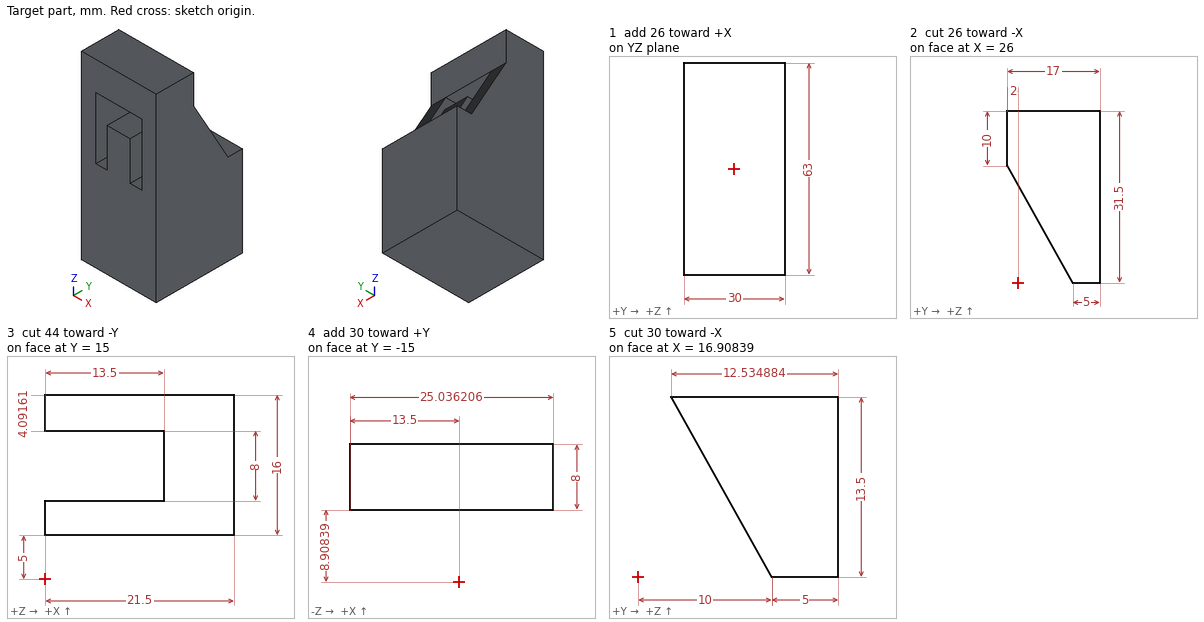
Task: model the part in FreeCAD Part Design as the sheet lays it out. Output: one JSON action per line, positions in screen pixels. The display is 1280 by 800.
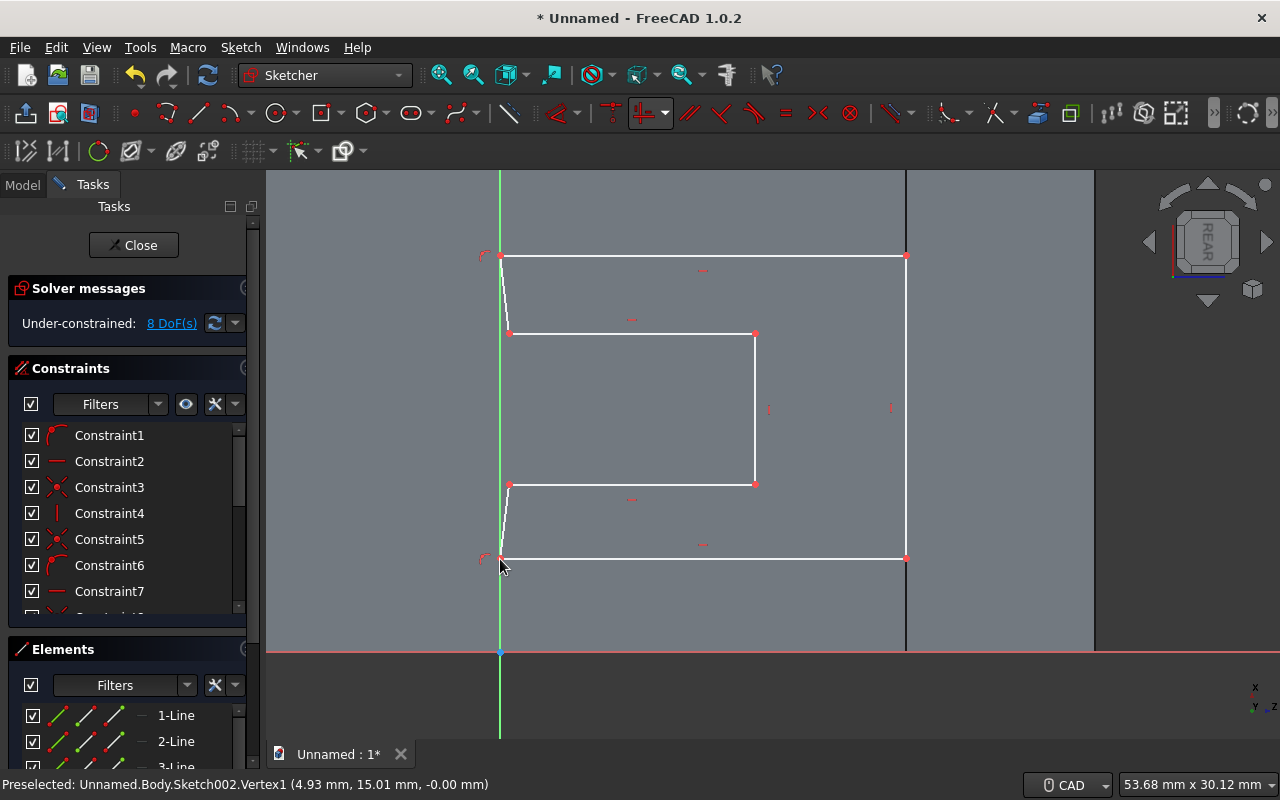
{"action": "left_click", "coordinate": [503, 279]}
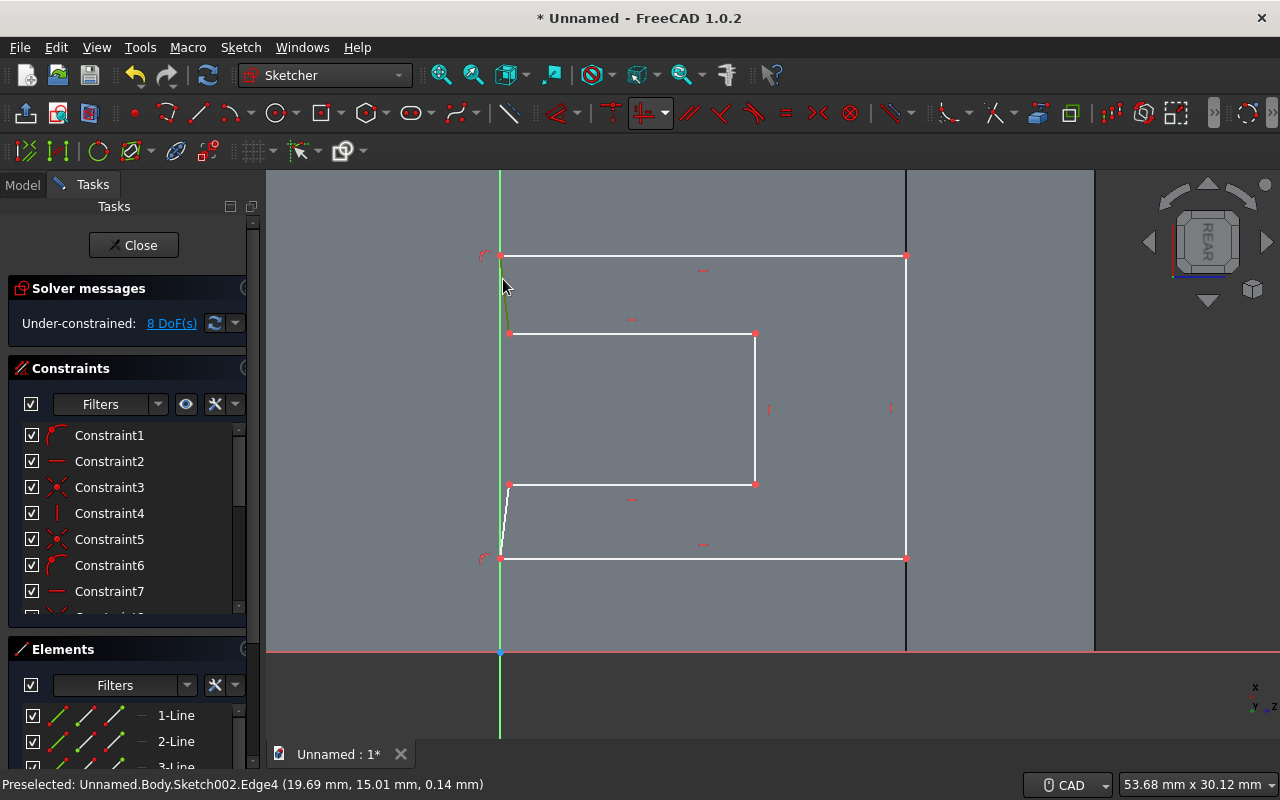
{"action": "key", "text": "v"}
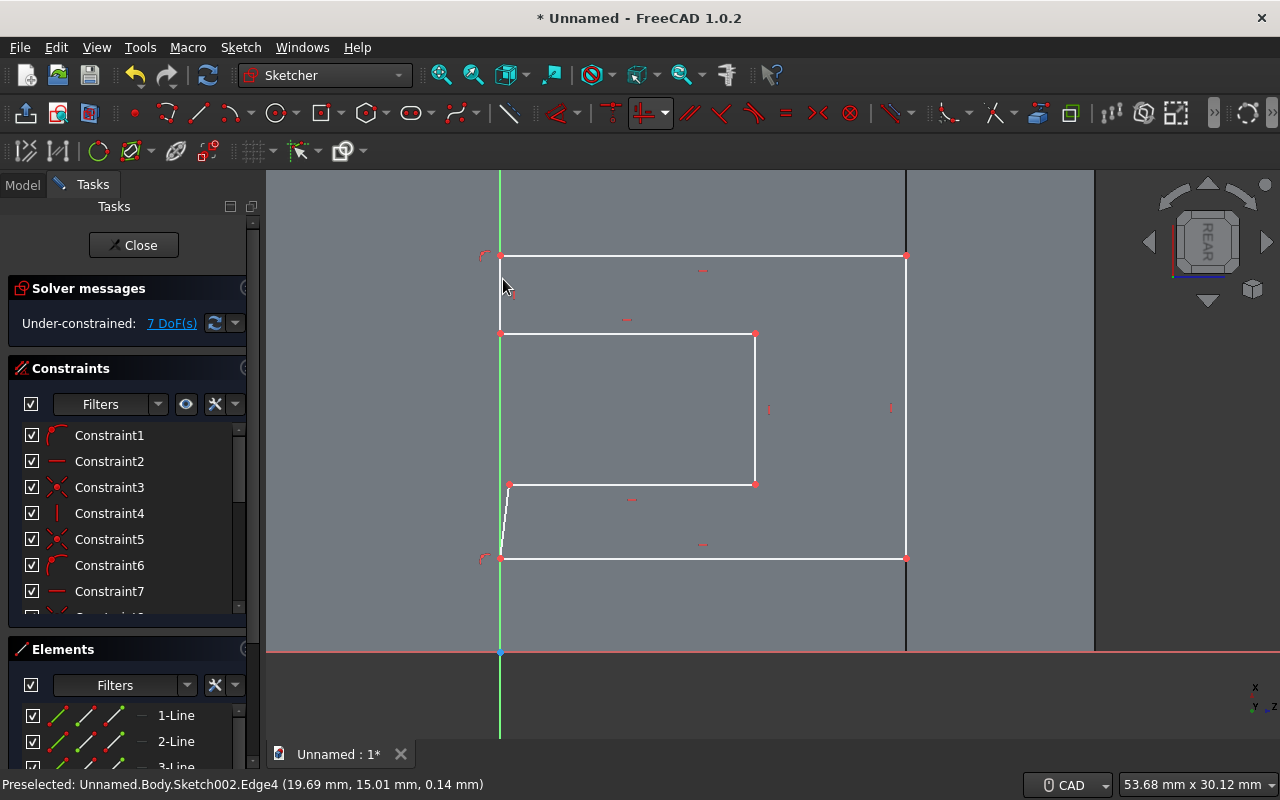
{"action": "left_click", "coordinate": [503, 537]}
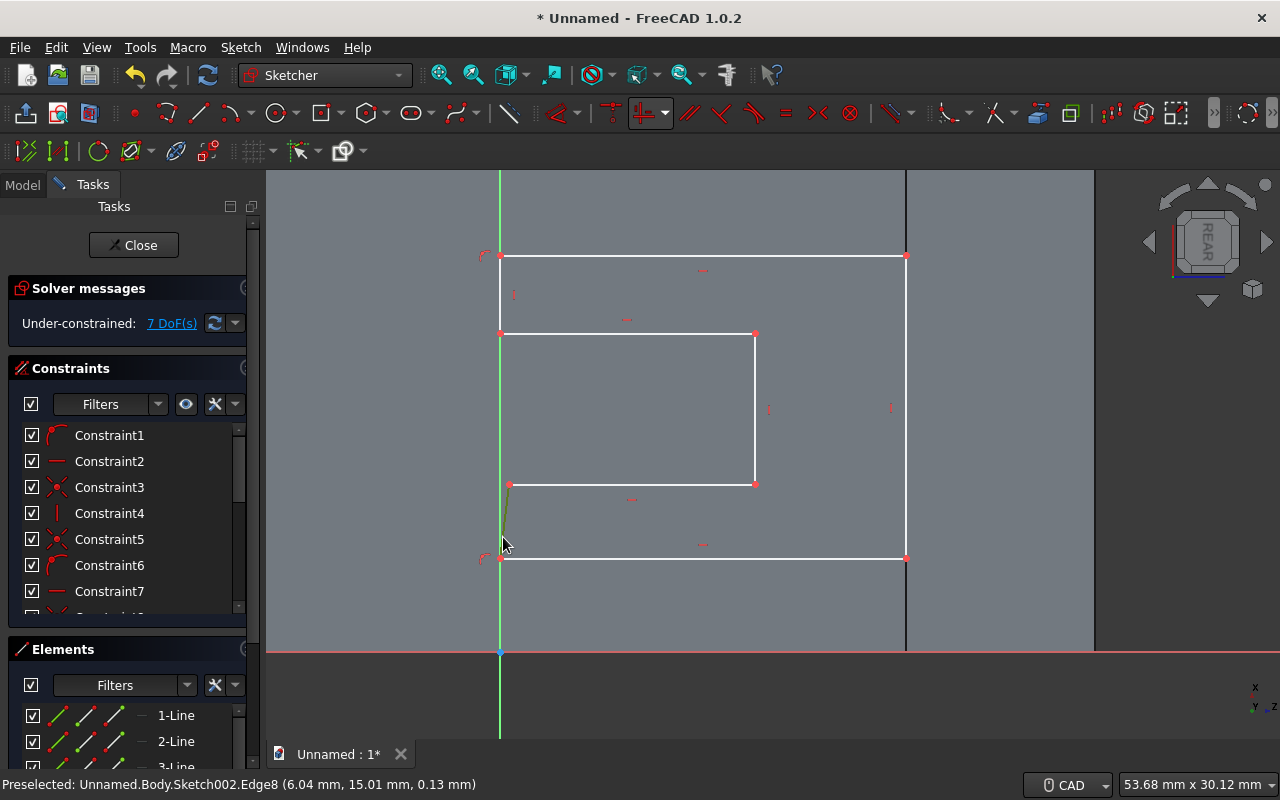
{"action": "key", "text": "v"}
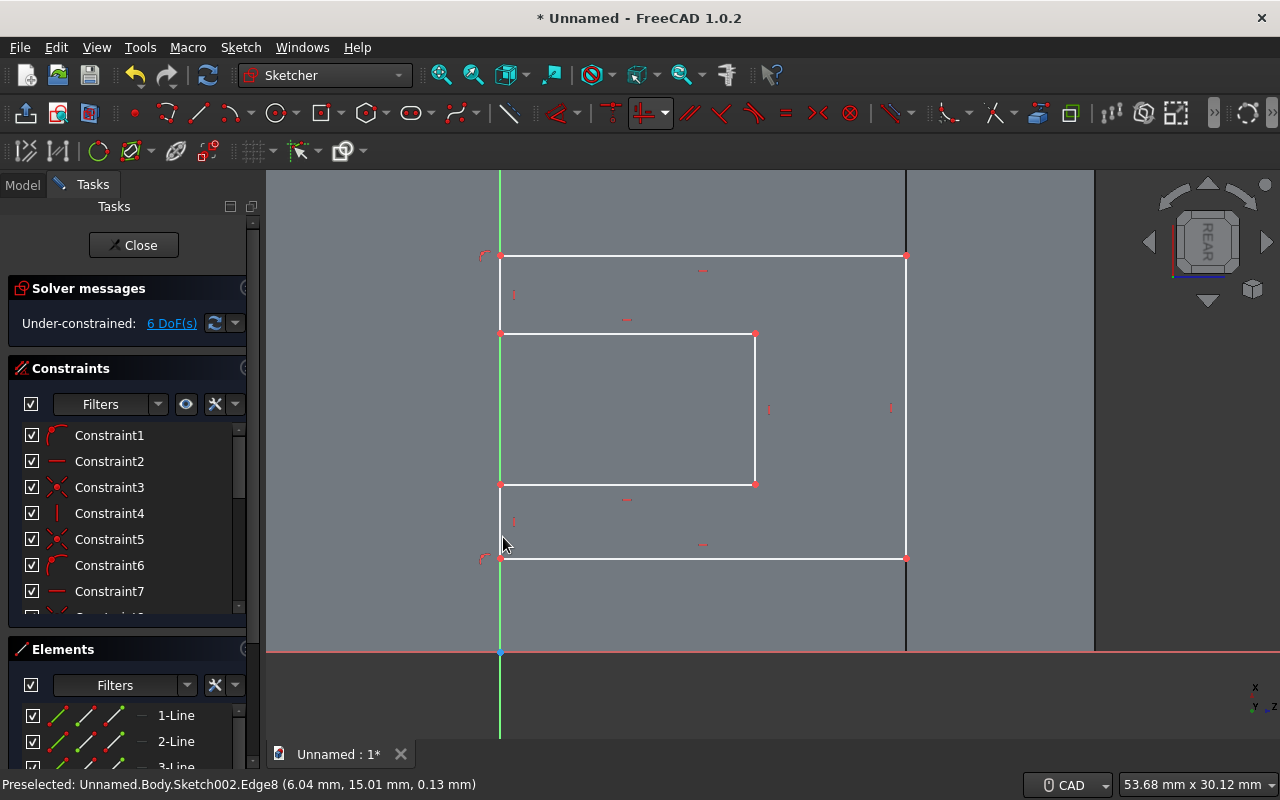
{"action": "key", "text": "d"}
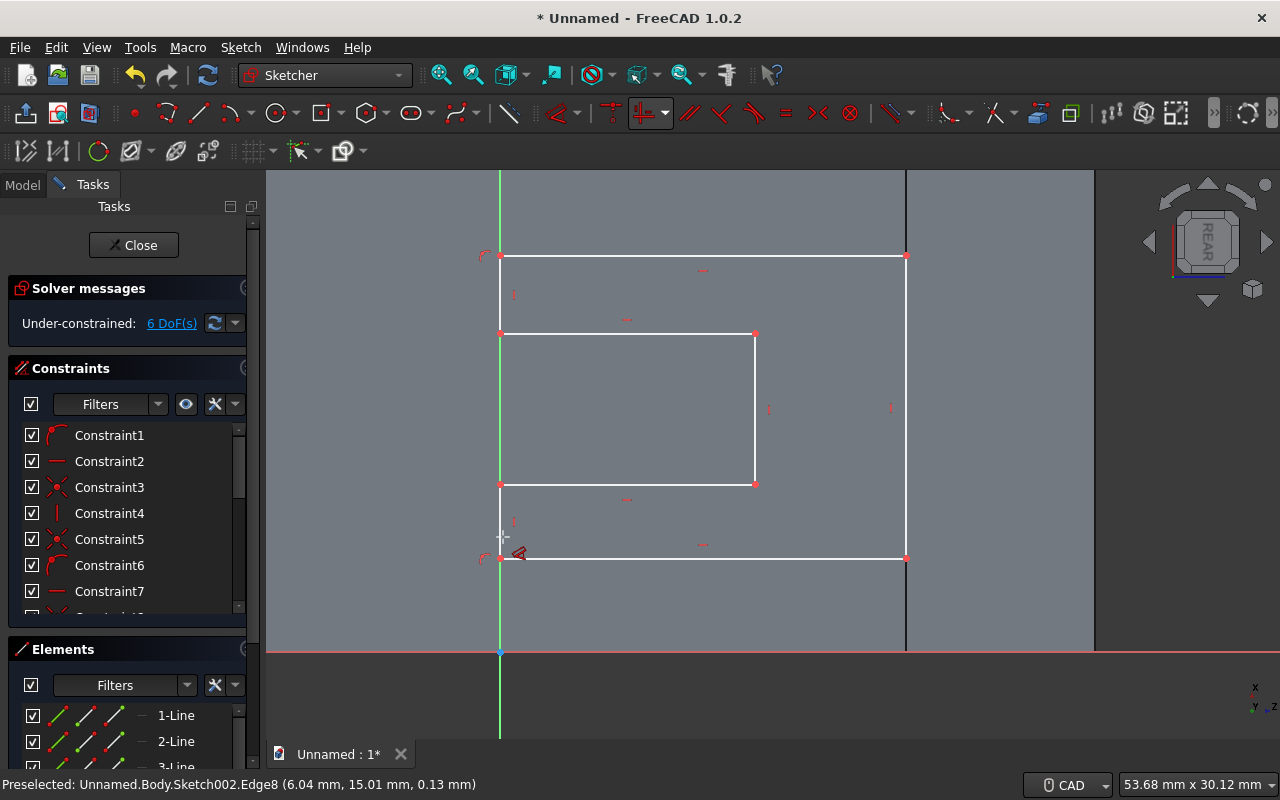
{"action": "left_click", "coordinate": [755, 379]}
{"action": "left_click", "coordinate": [789, 409]}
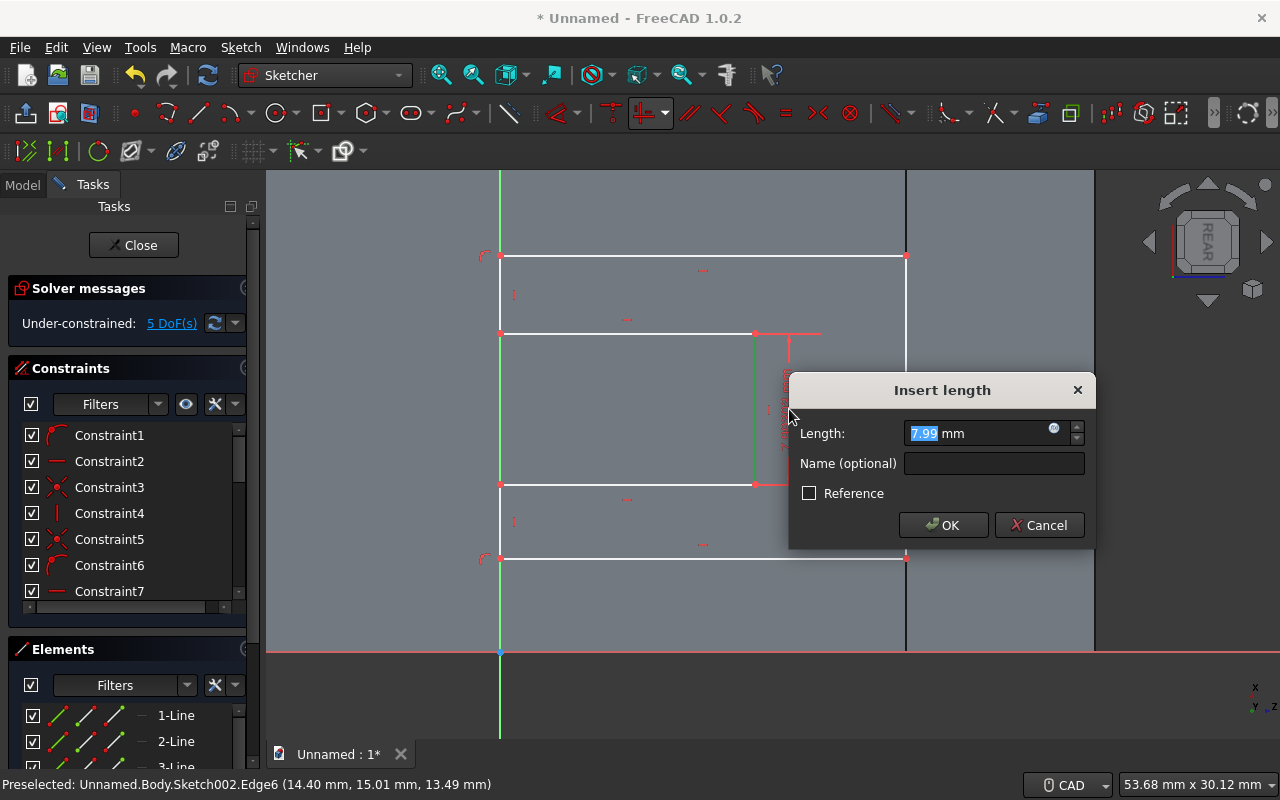
{"action": "type", "text": "8"}
{"action": "key", "text": "Return"}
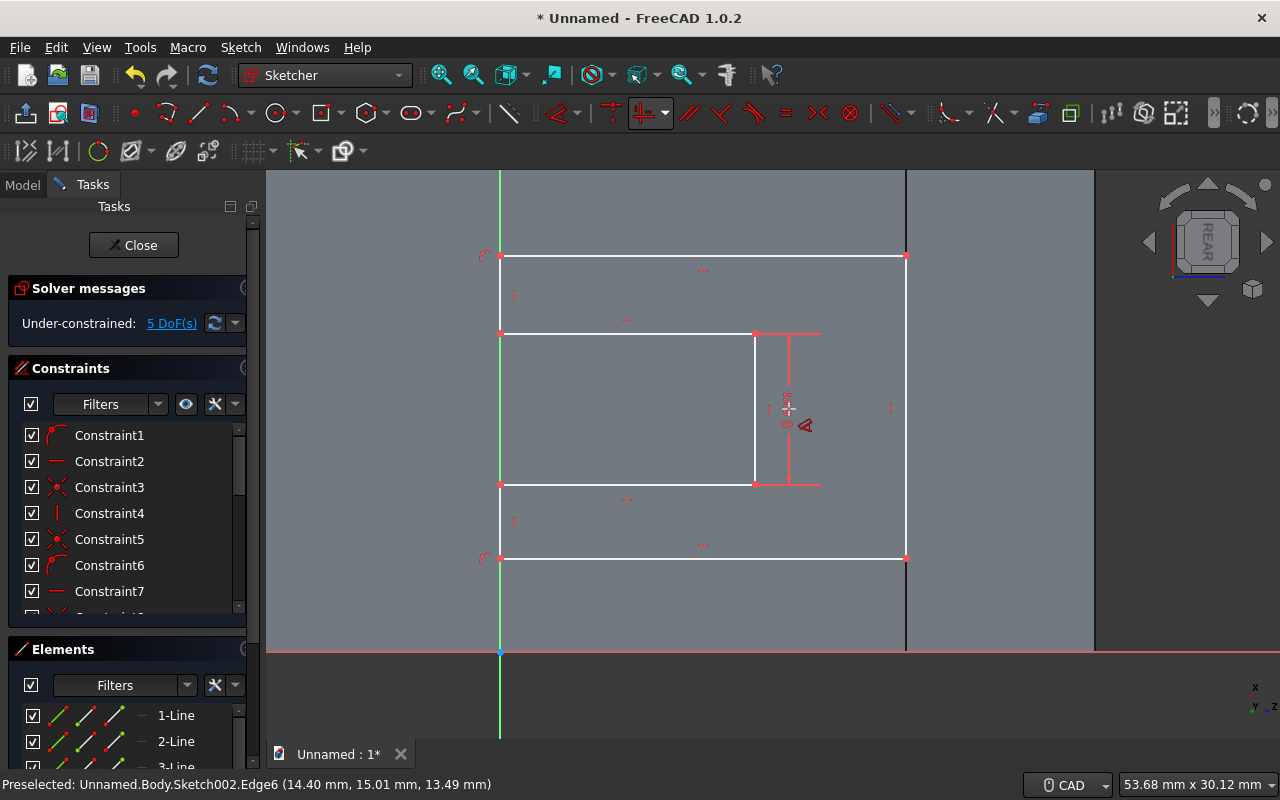
{"action": "left_click", "coordinate": [906, 468]}
{"action": "left_click", "coordinate": [940, 408]}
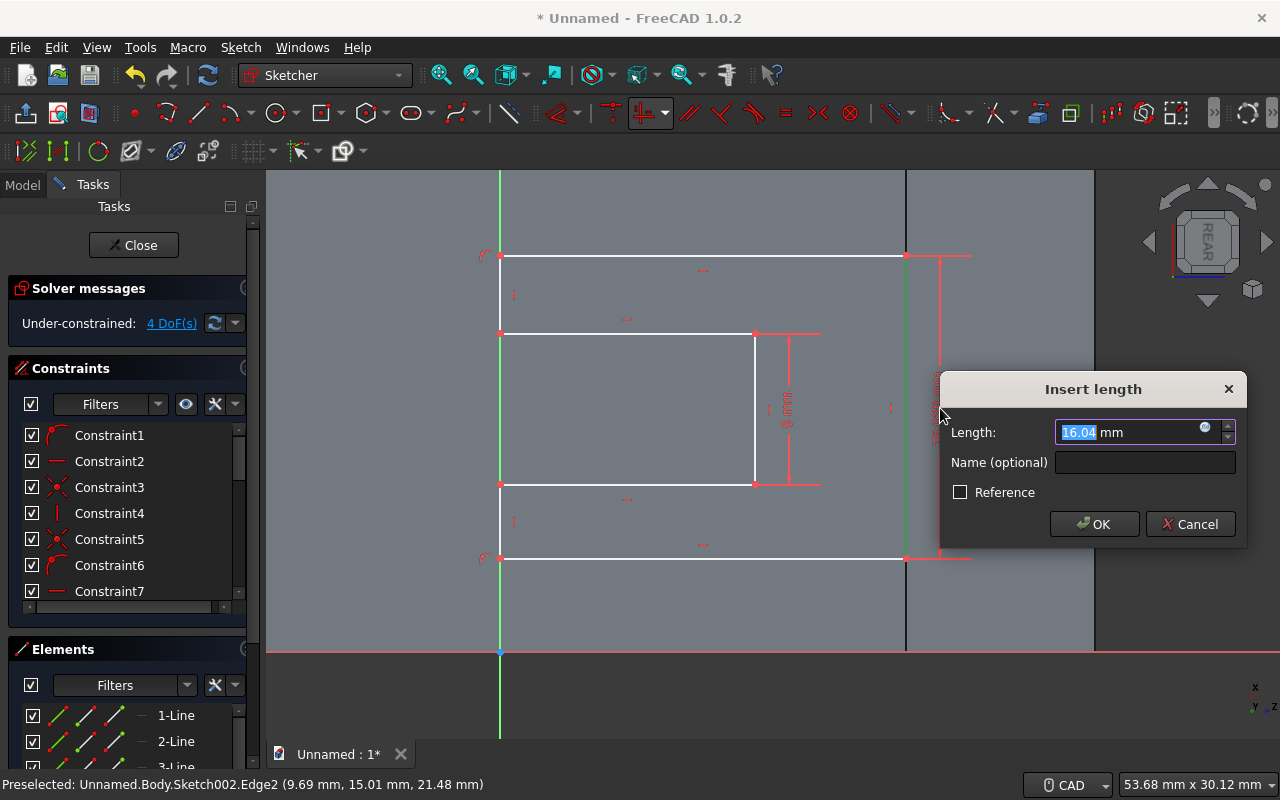
{"action": "type", "text": "16"}
{"action": "key", "text": "Return"}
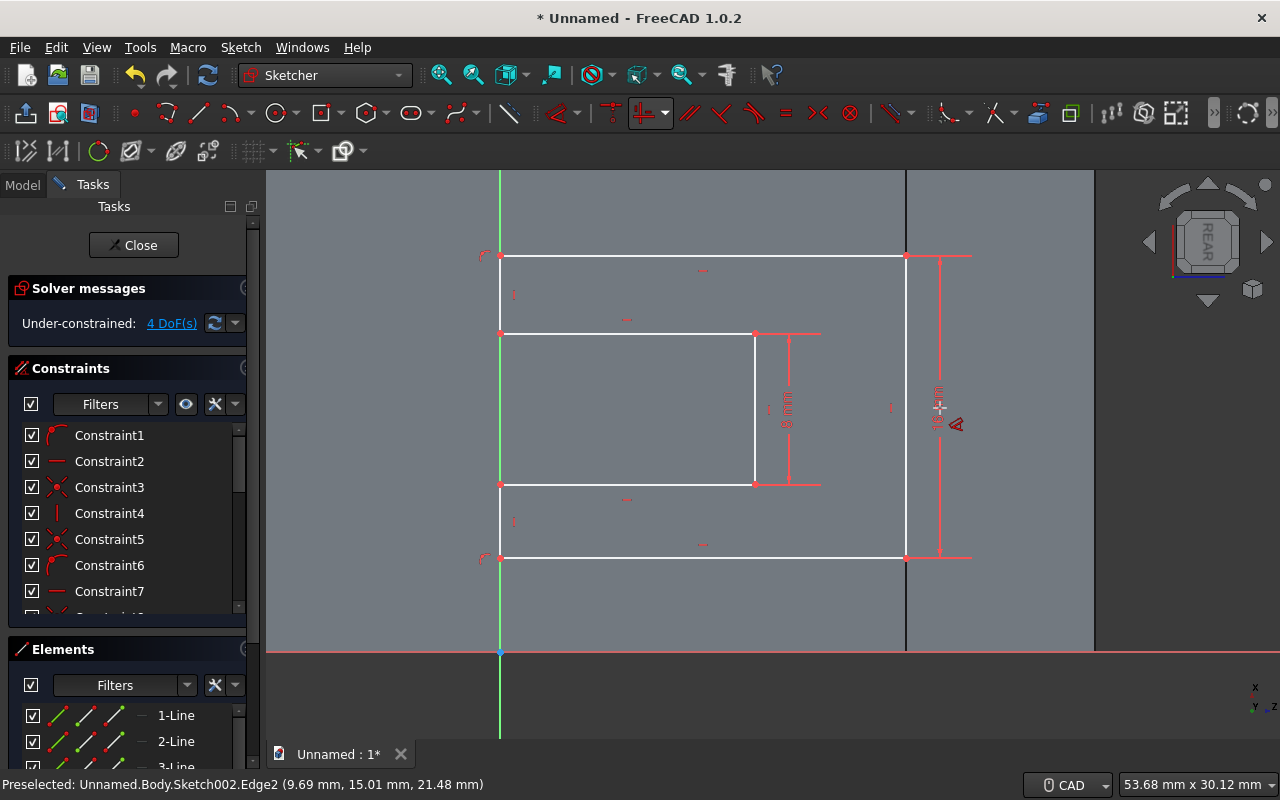
{"action": "left_click", "coordinate": [500, 558]}
{"action": "left_click", "coordinate": [466, 605]}